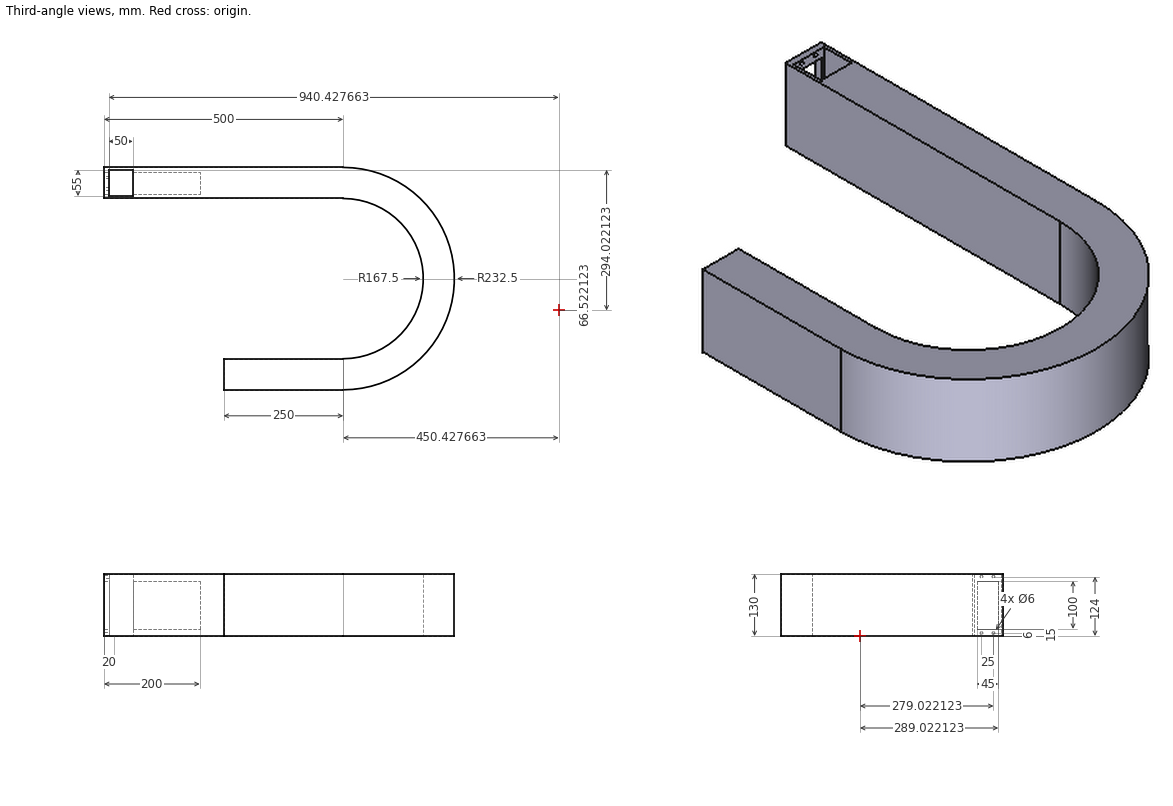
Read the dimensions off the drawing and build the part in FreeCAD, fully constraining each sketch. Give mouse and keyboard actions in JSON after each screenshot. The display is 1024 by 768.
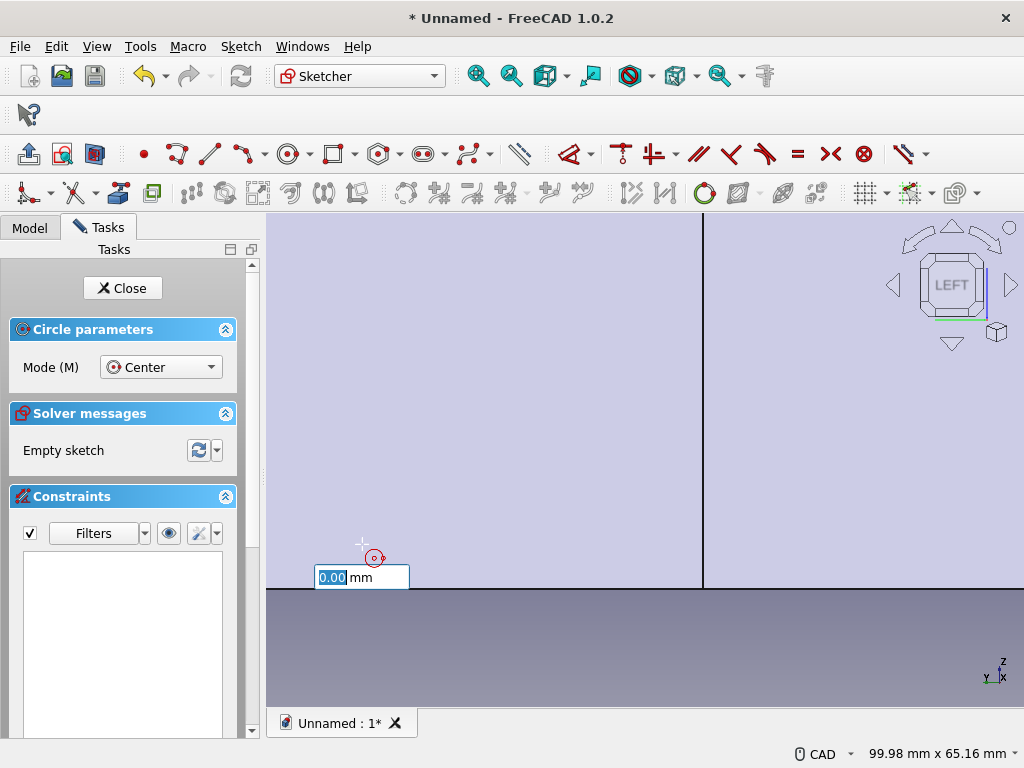
{"action": "scroll", "coordinate": [366, 549], "scroll_direction": "down", "scroll_amount": 8}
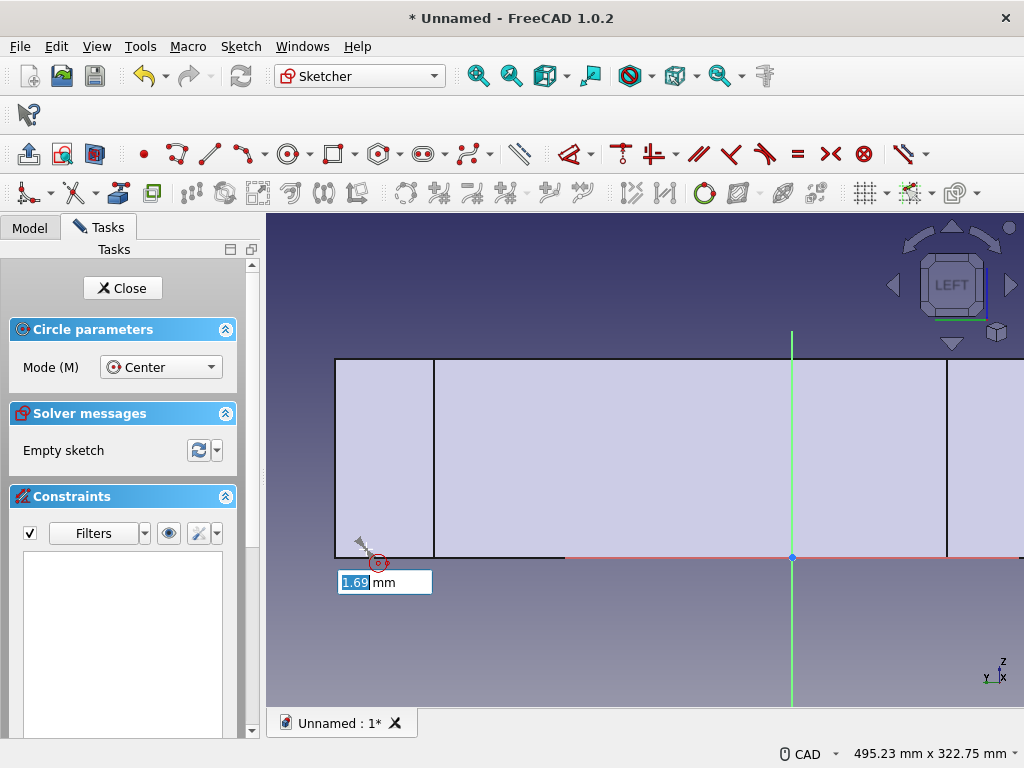
{"action": "scroll", "coordinate": [368, 545], "scroll_direction": "up", "scroll_amount": 2}
{"action": "mouse_move", "coordinate": [369, 545]}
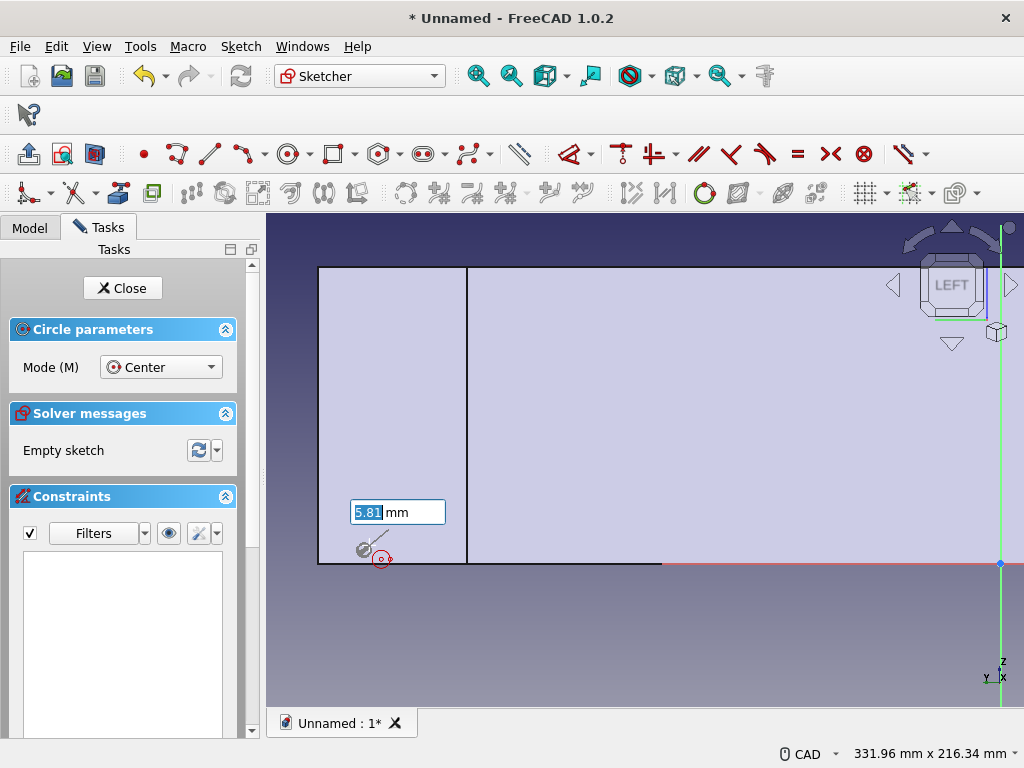
{"action": "type", "text": "6"}
{"action": "key", "text": "Return"}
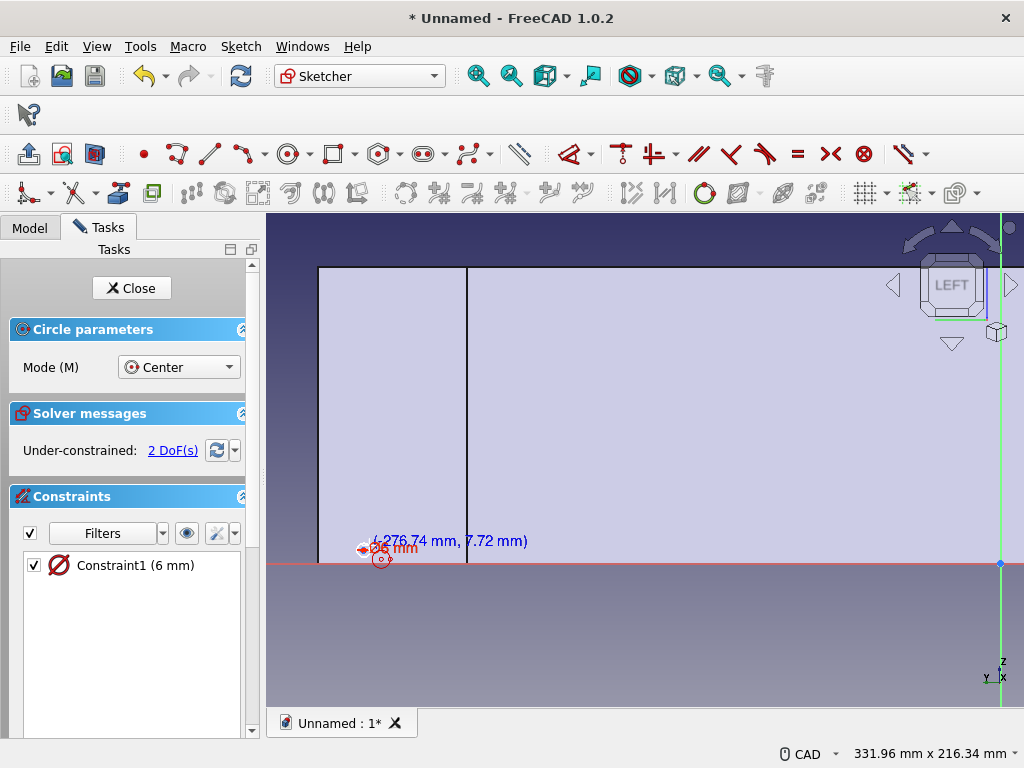
{"action": "scroll", "coordinate": [421, 550], "scroll_direction": "up", "scroll_amount": 6}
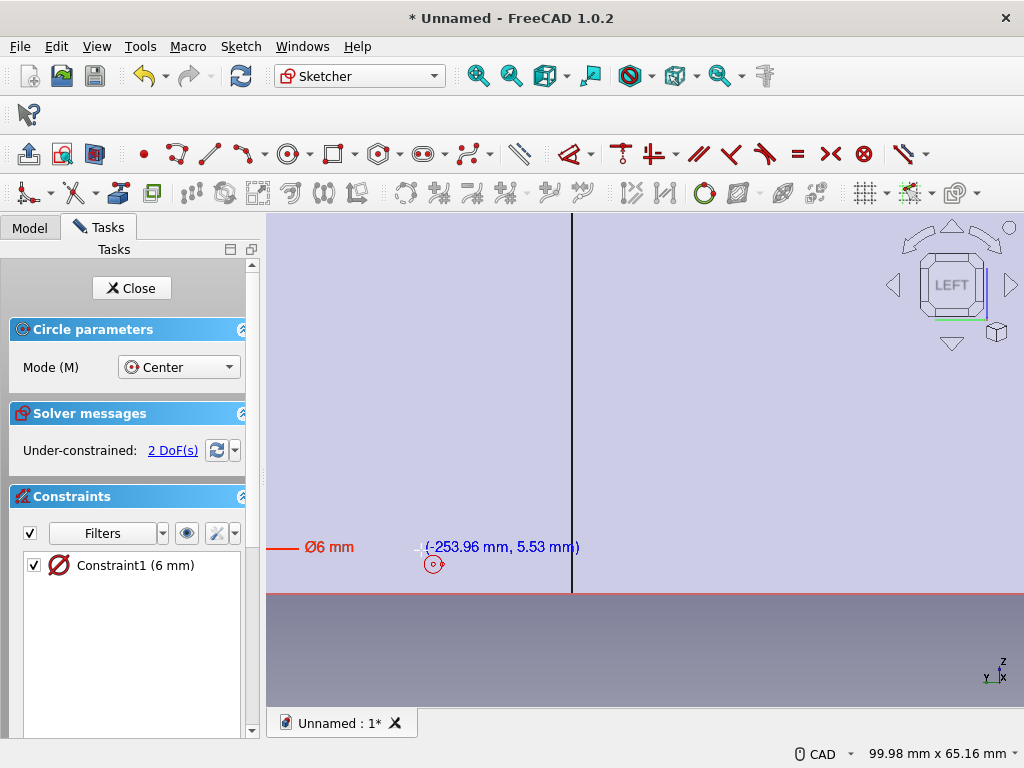
{"action": "left_click", "coordinate": [420, 548]}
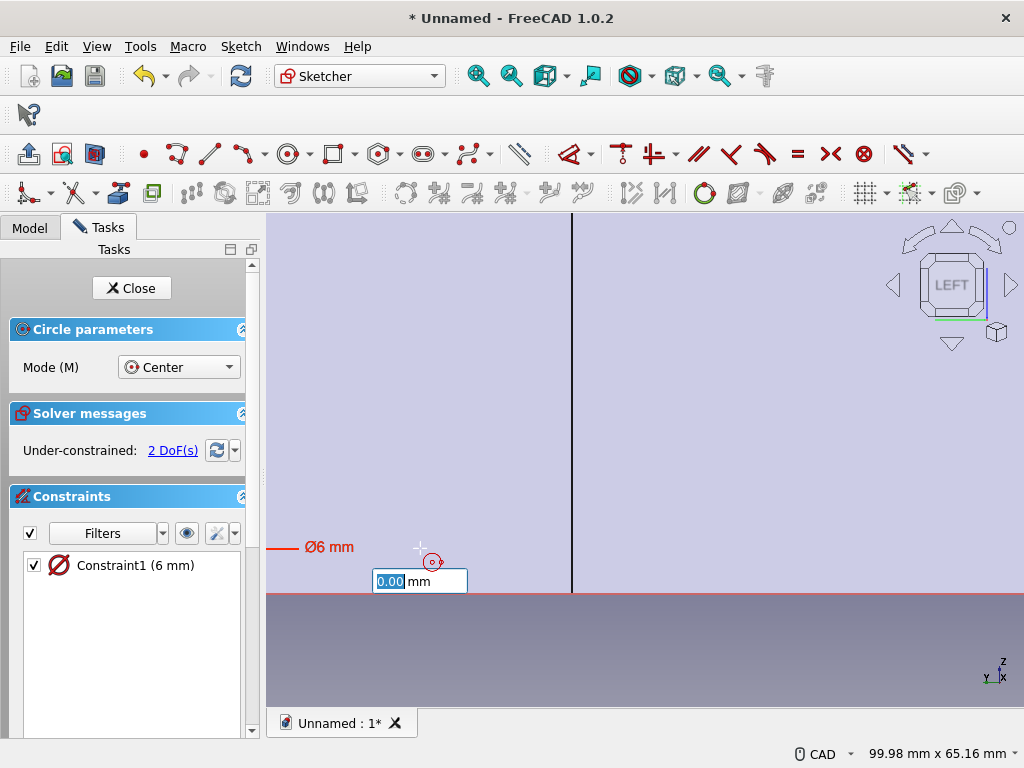
{"action": "scroll", "coordinate": [399, 548], "scroll_direction": "down", "scroll_amount": 8}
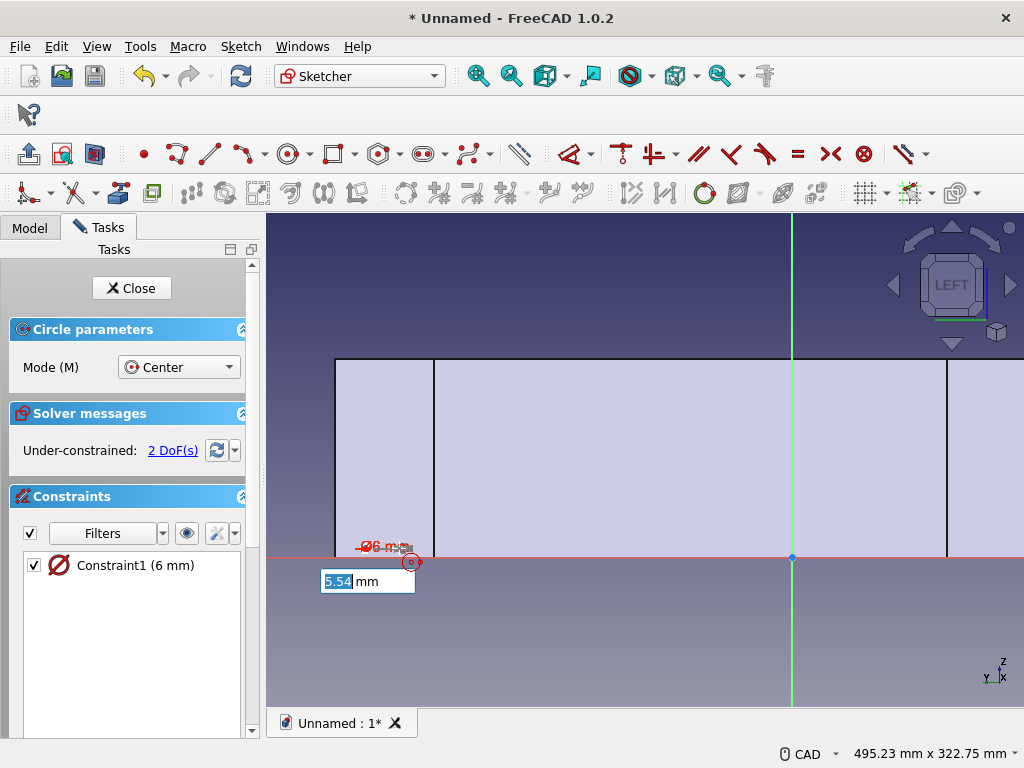
{"action": "scroll", "coordinate": [407, 545], "scroll_direction": "up", "scroll_amount": 2}
{"action": "mouse_move", "coordinate": [406, 545]}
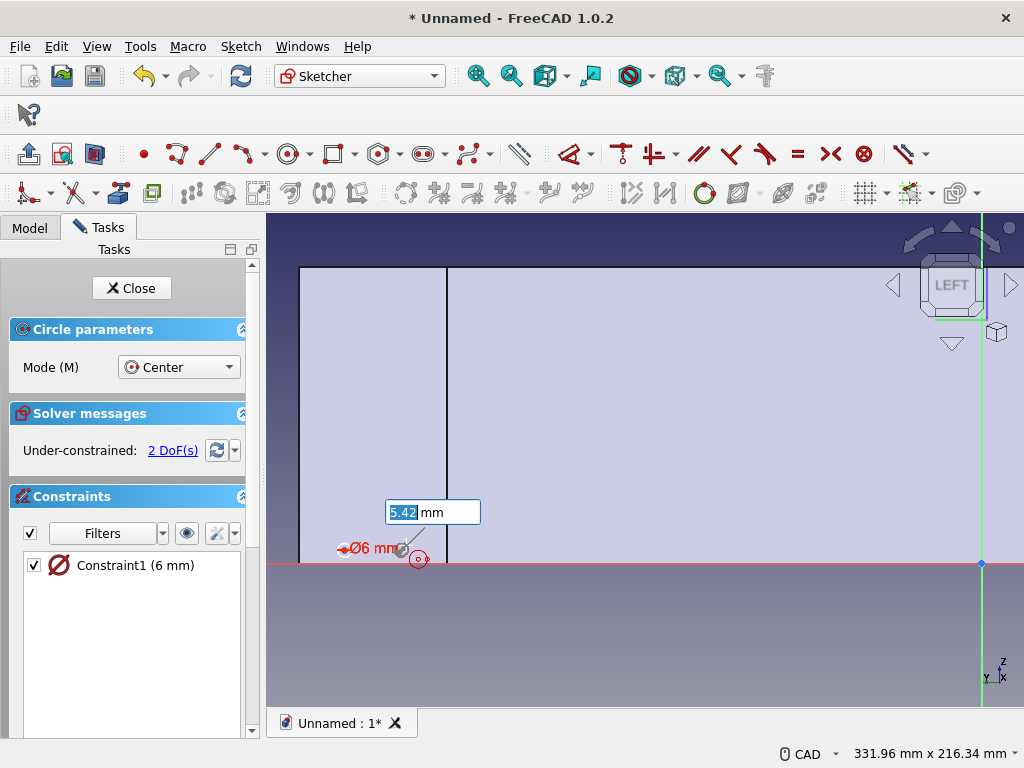
{"action": "type", "text": "6"}
{"action": "key", "text": "Return"}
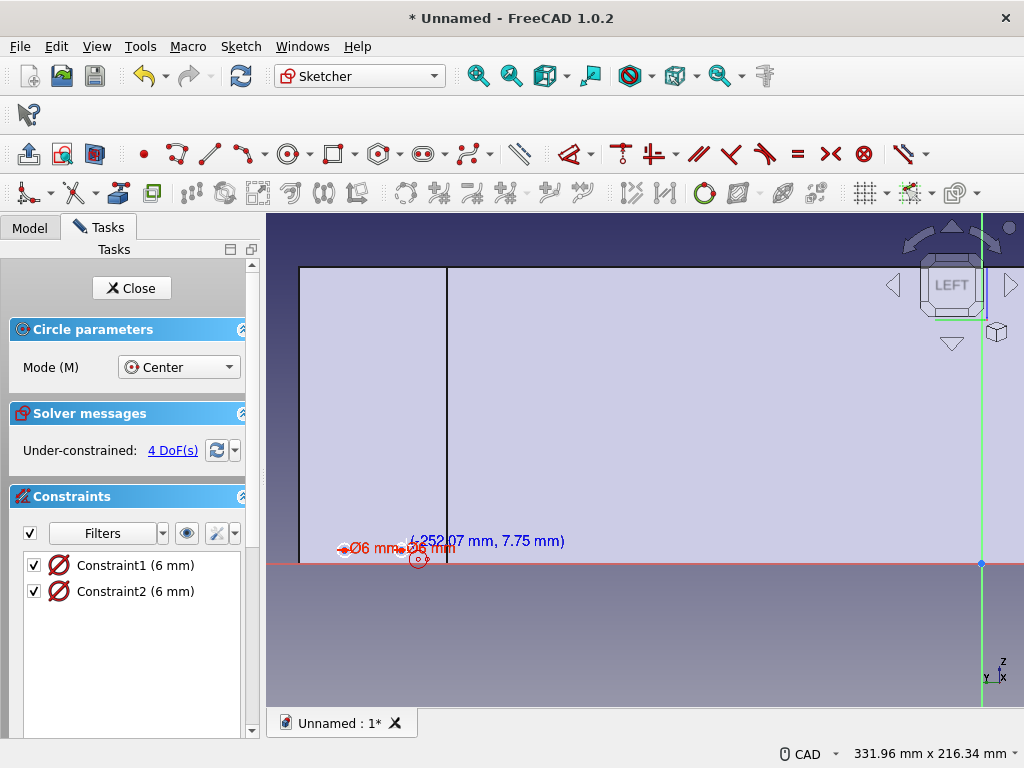
{"action": "scroll", "coordinate": [344, 281], "scroll_direction": "up", "scroll_amount": 6}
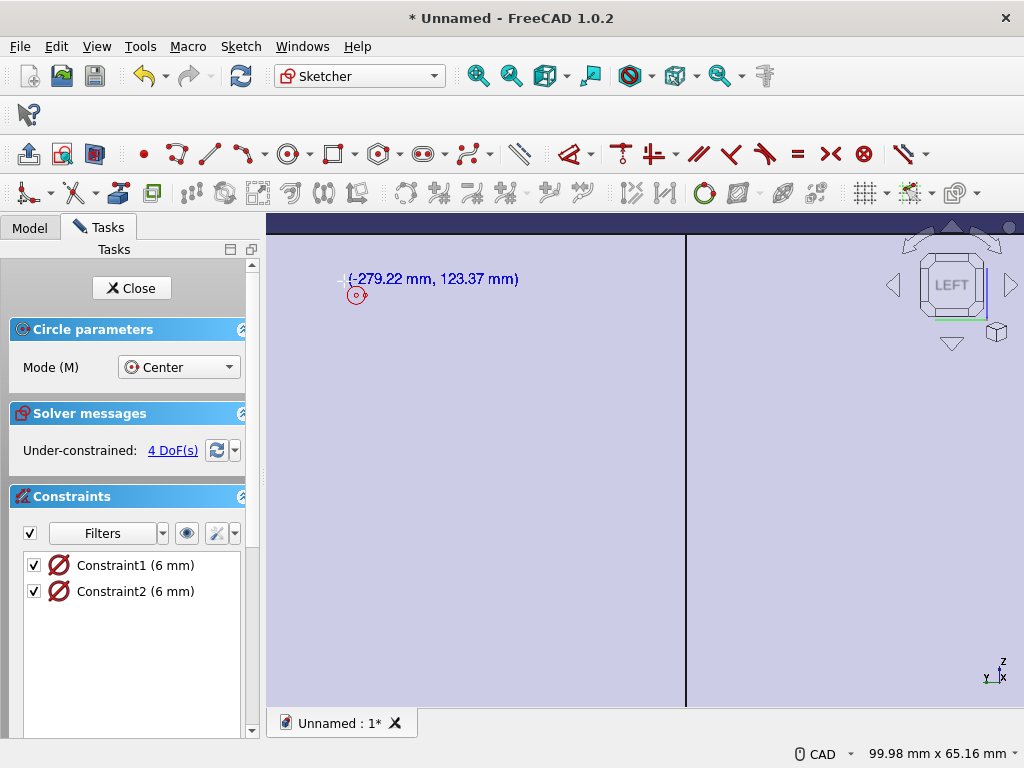
{"action": "scroll", "coordinate": [370, 390], "scroll_direction": "down", "scroll_amount": 8}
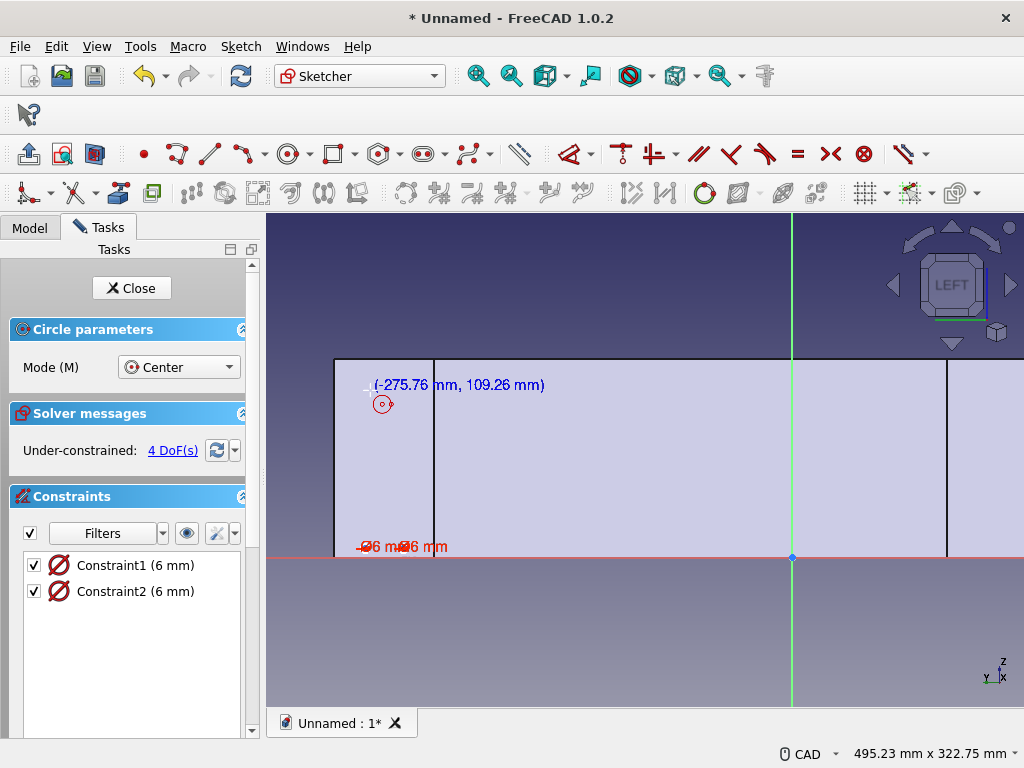
{"action": "left_click", "coordinate": [365, 368]}
{"action": "mouse_move", "coordinate": [368, 365]}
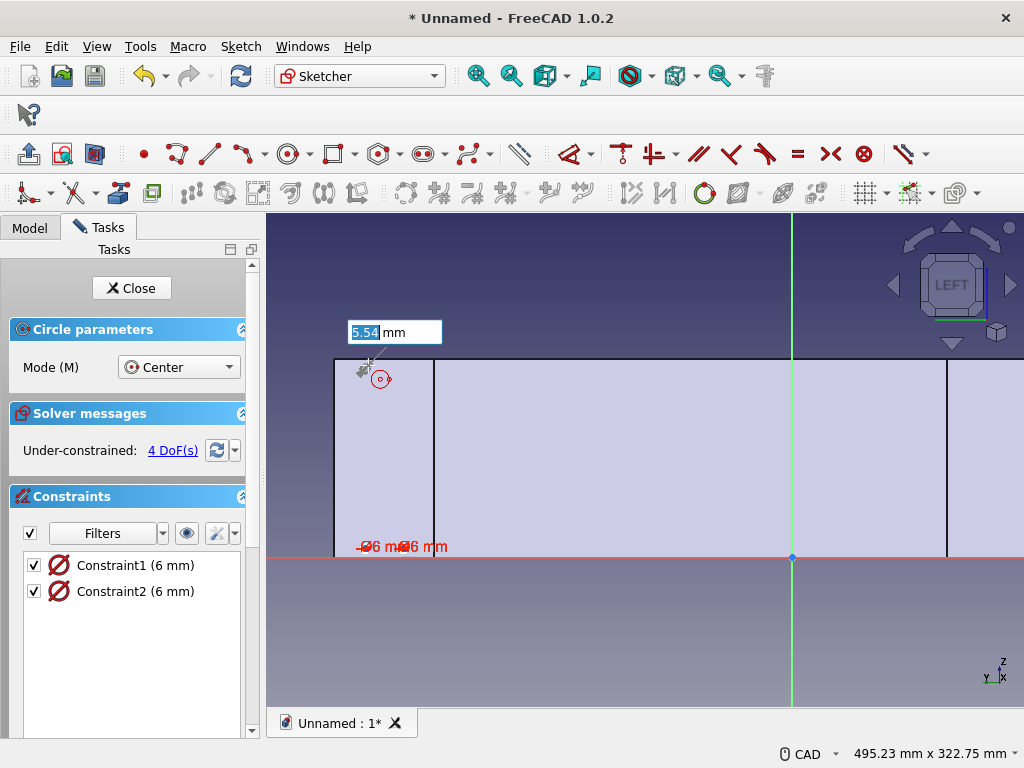
{"action": "type", "text": "6"}
{"action": "key", "text": "Return"}